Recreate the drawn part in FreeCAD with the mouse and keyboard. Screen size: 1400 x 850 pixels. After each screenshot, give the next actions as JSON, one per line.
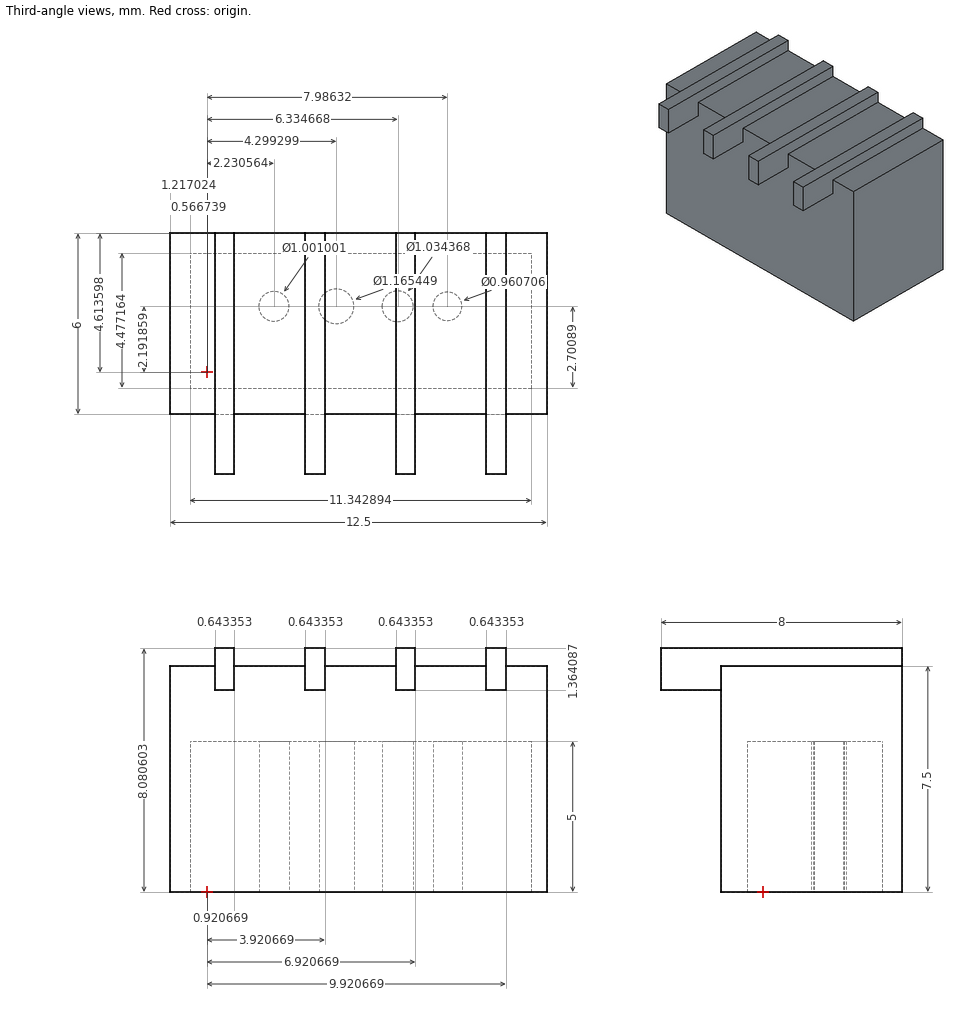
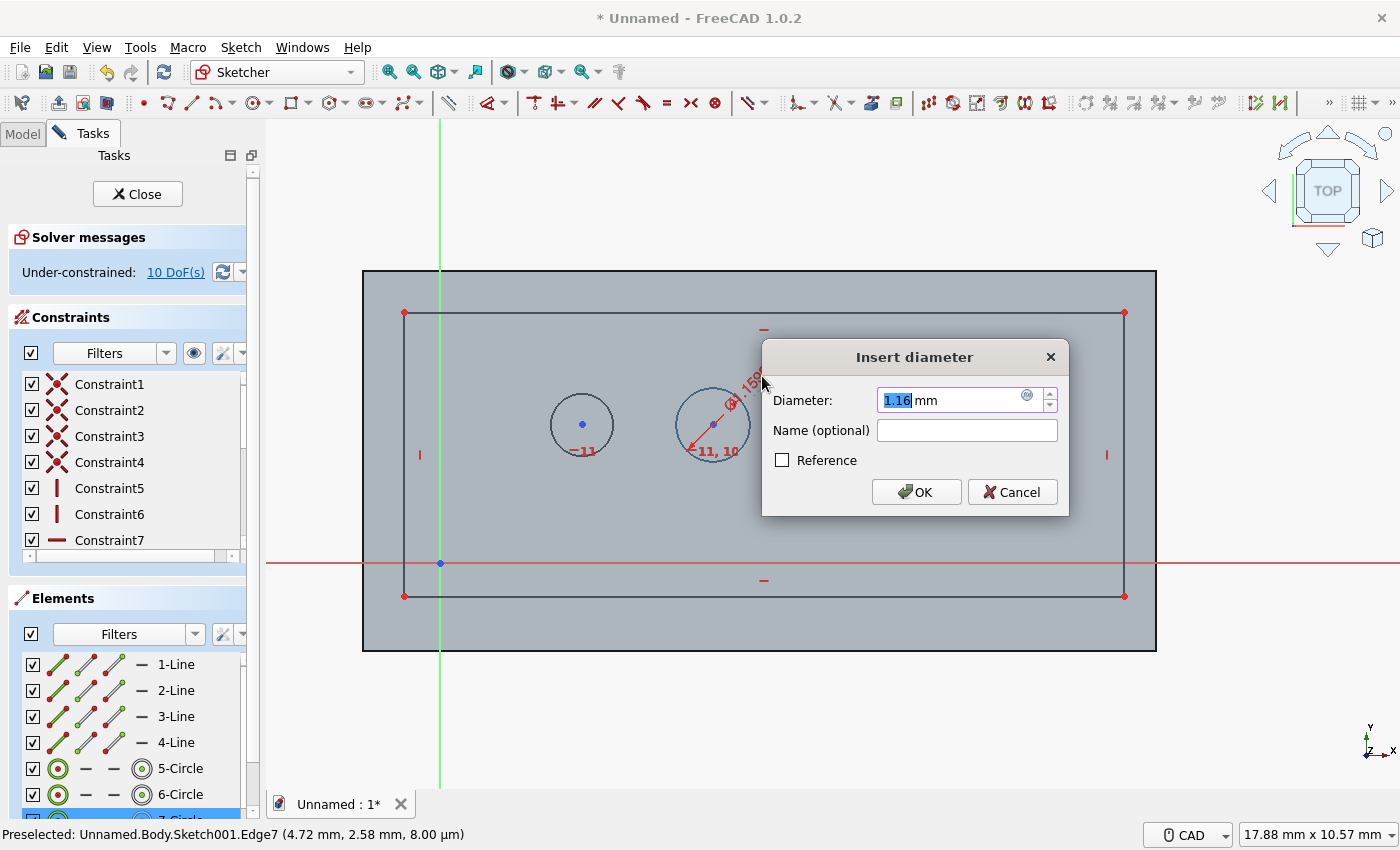
{"action": "type", "text": "1.165449"}
{"action": "key", "text": "Return"}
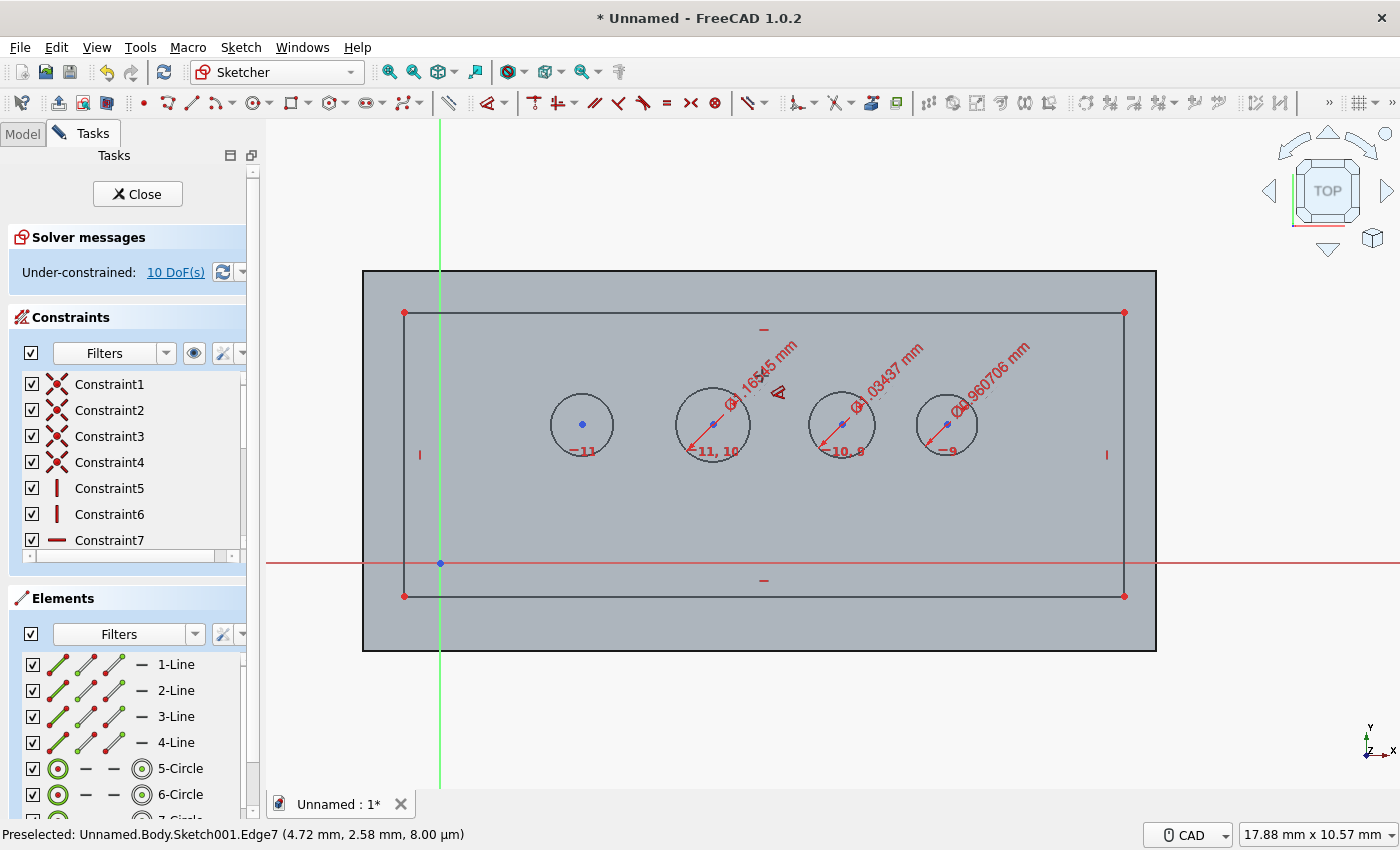
{"action": "left_click", "coordinate": [604, 403]}
{"action": "left_click", "coordinate": [627, 380]}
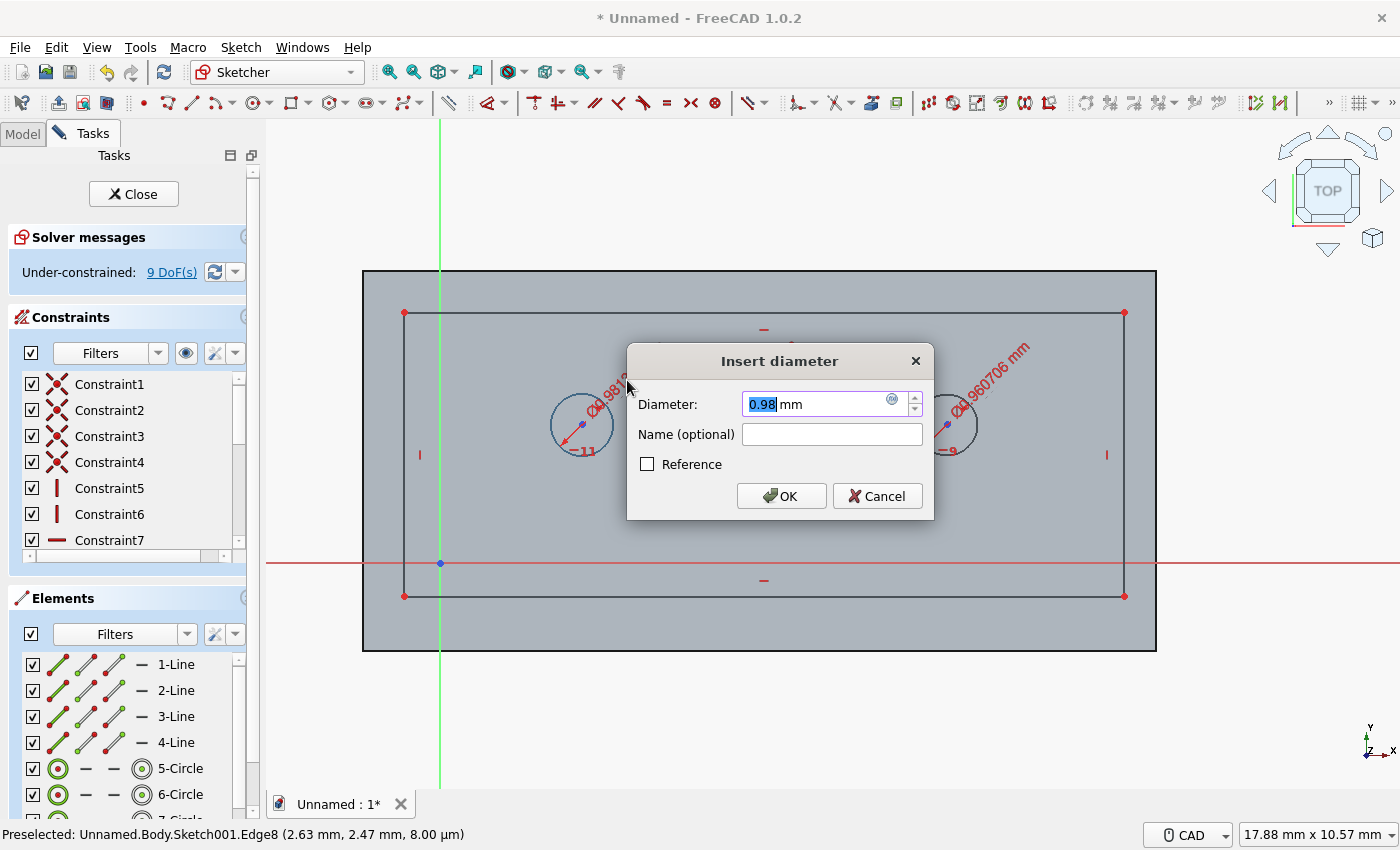
{"action": "type", "text": "1.001001"}
{"action": "key", "text": "Return"}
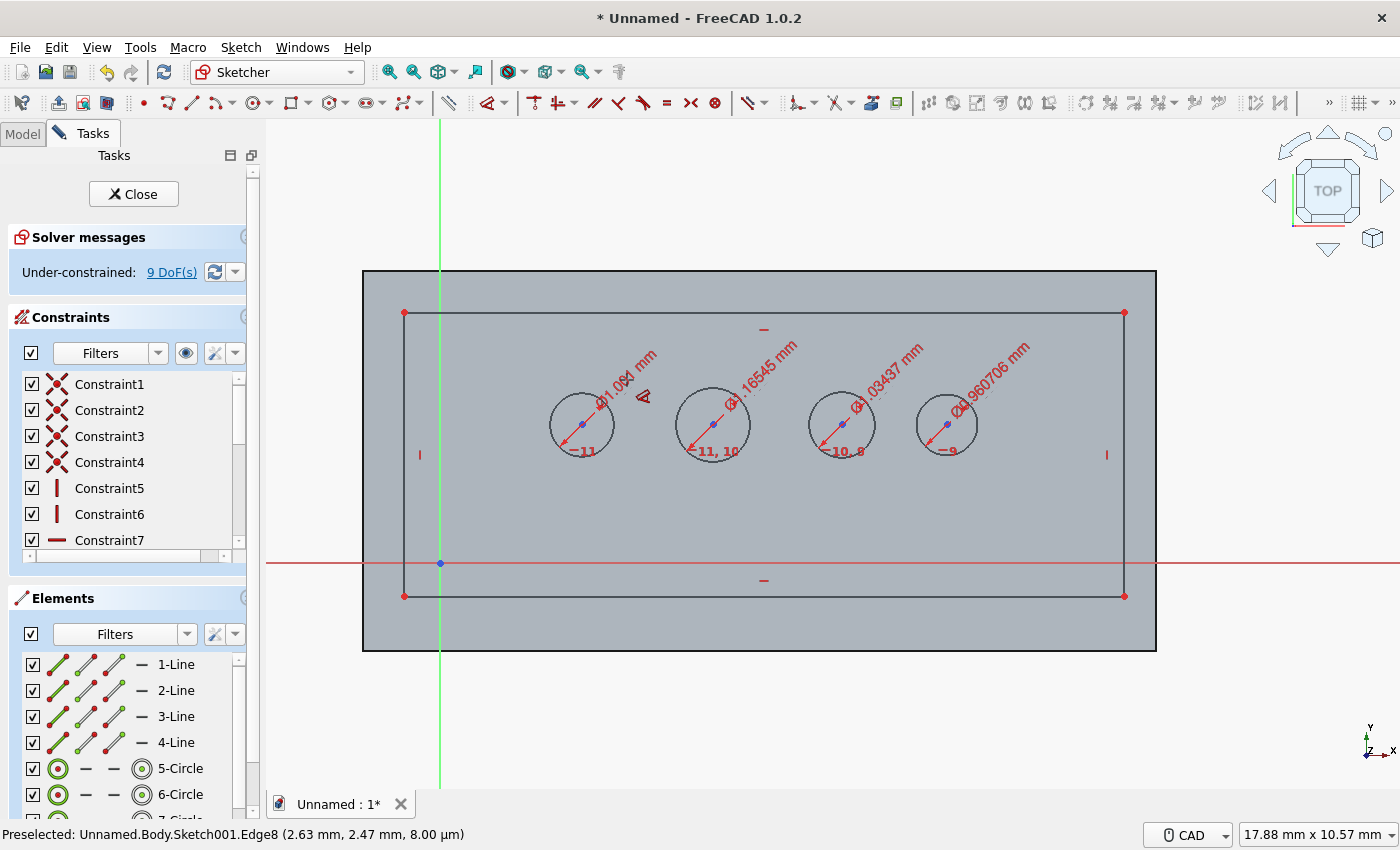
{"action": "left_click", "coordinate": [947, 425]}
{"action": "left_click", "coordinate": [516, 391]}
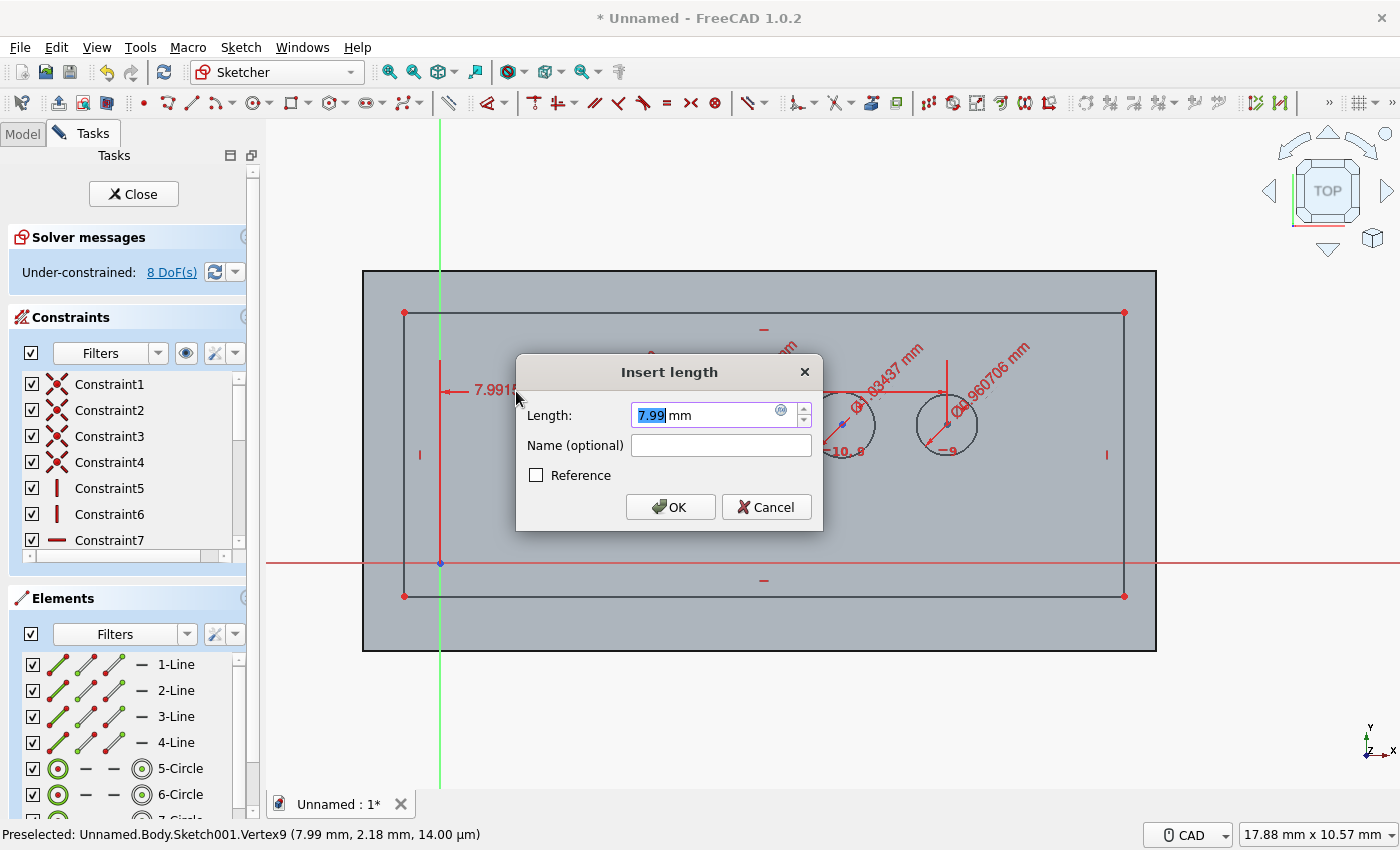
{"action": "type", "text": "7.98632"}
{"action": "key", "text": "Return"}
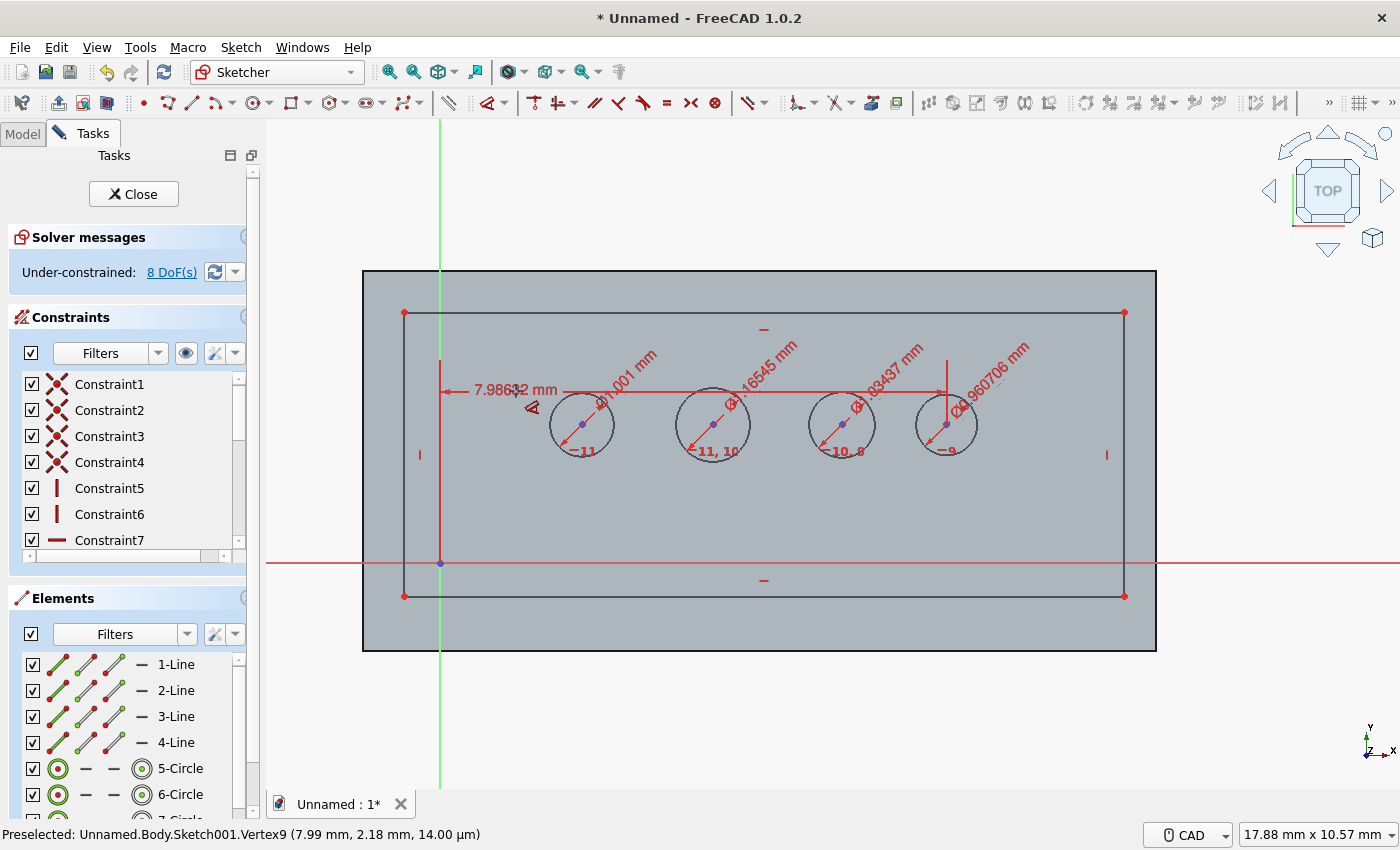
{"action": "left_click", "coordinate": [404, 398]}
{"action": "left_click", "coordinate": [370, 455]}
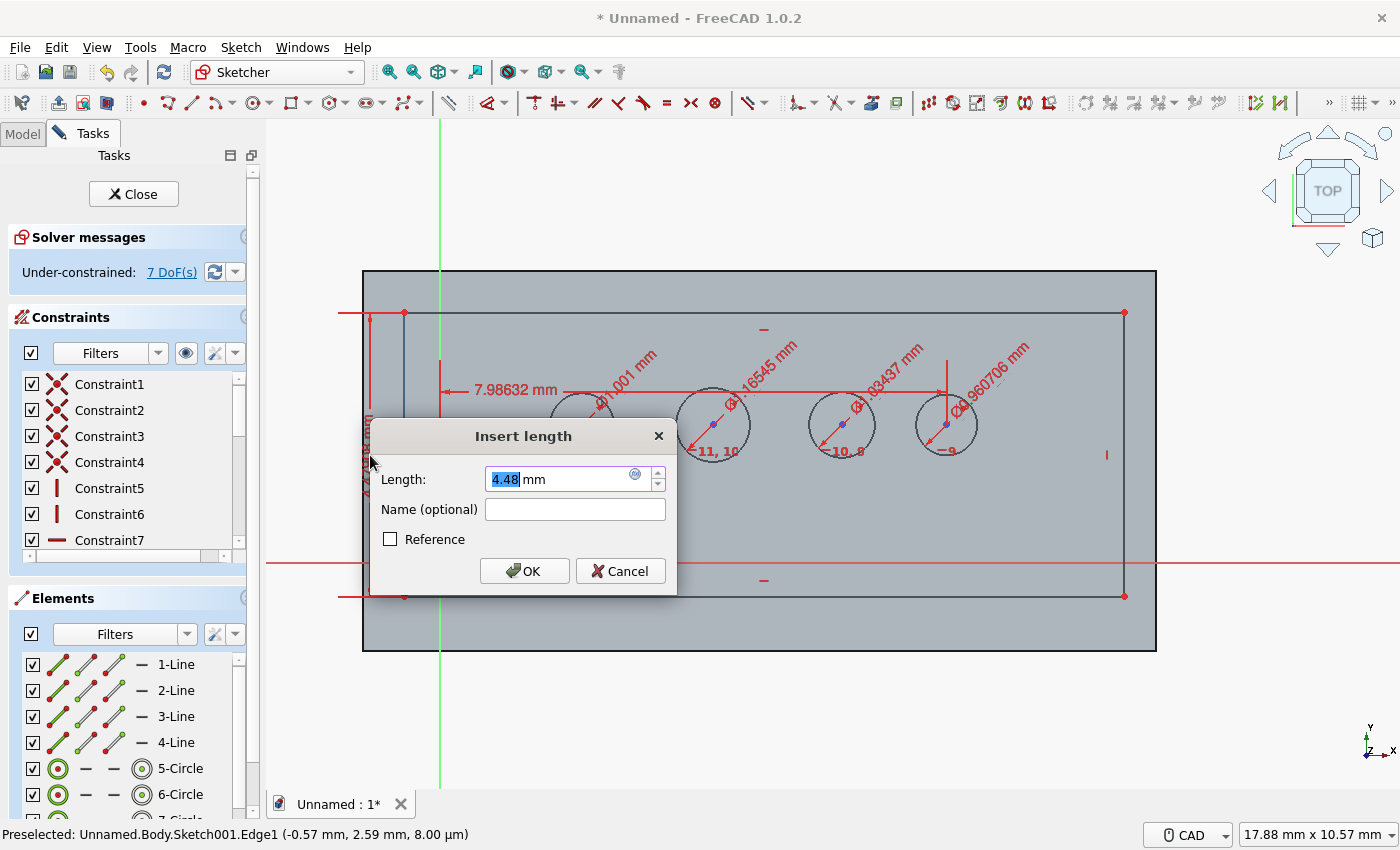
{"action": "type", "text": "4.477164"}
{"action": "key", "text": "Return"}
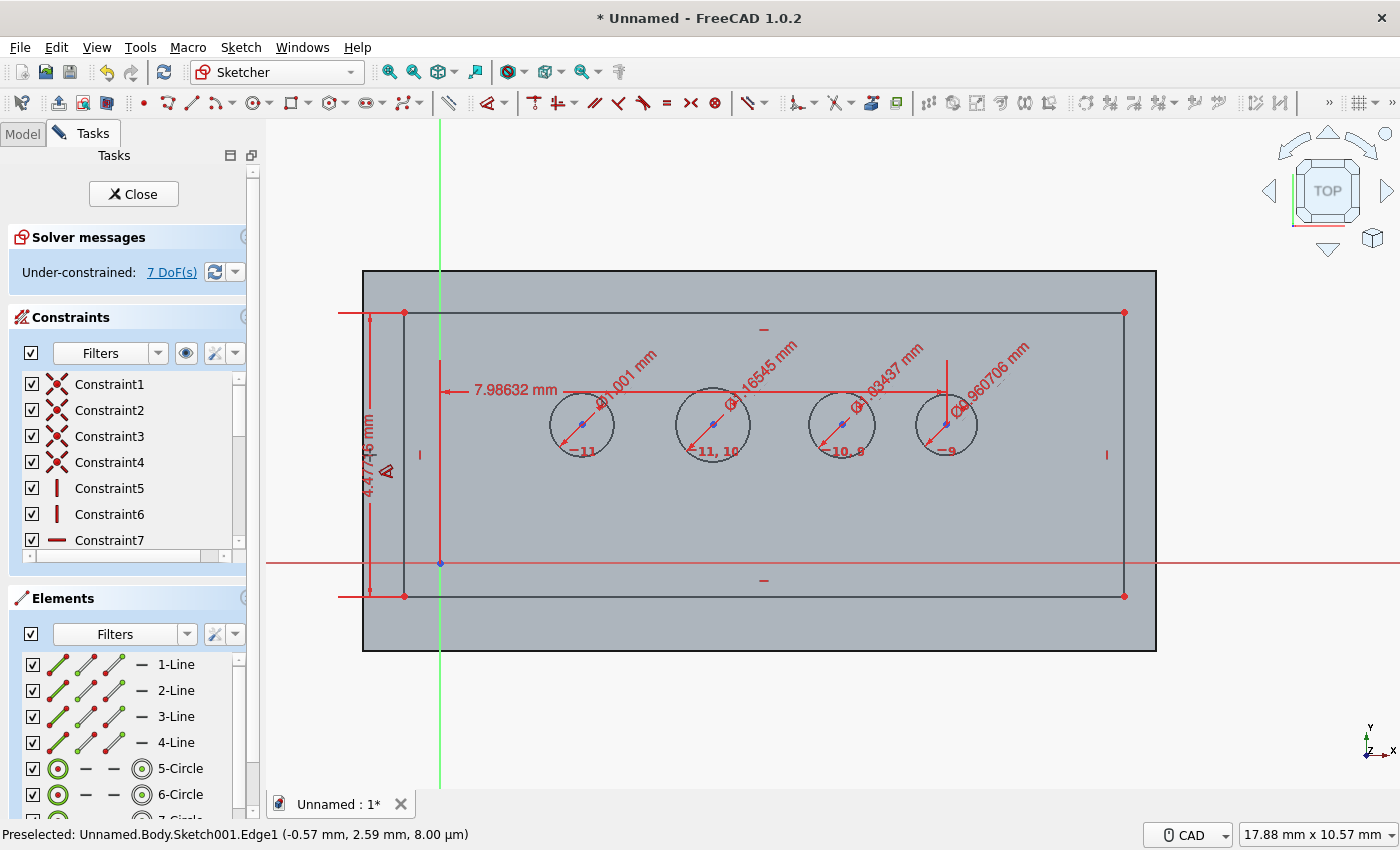
{"action": "left_click", "coordinate": [947, 425]}
{"action": "left_click", "coordinate": [981, 494]}